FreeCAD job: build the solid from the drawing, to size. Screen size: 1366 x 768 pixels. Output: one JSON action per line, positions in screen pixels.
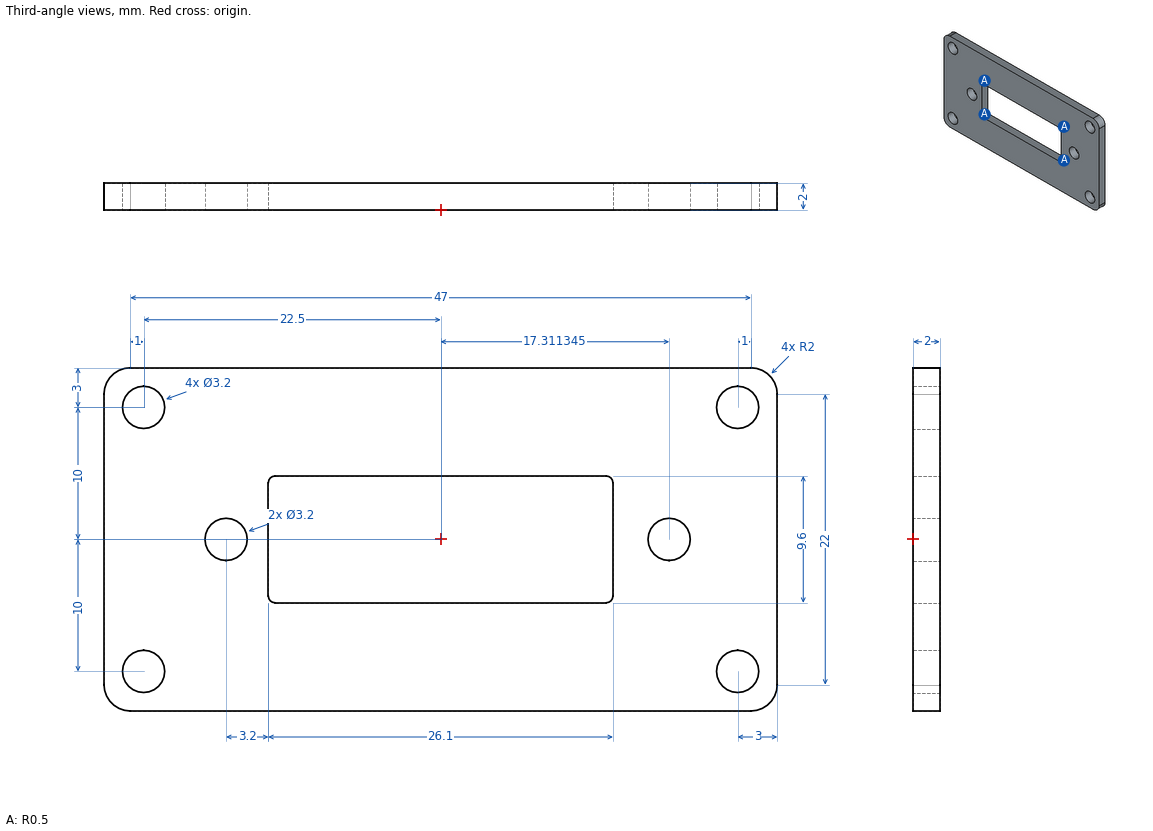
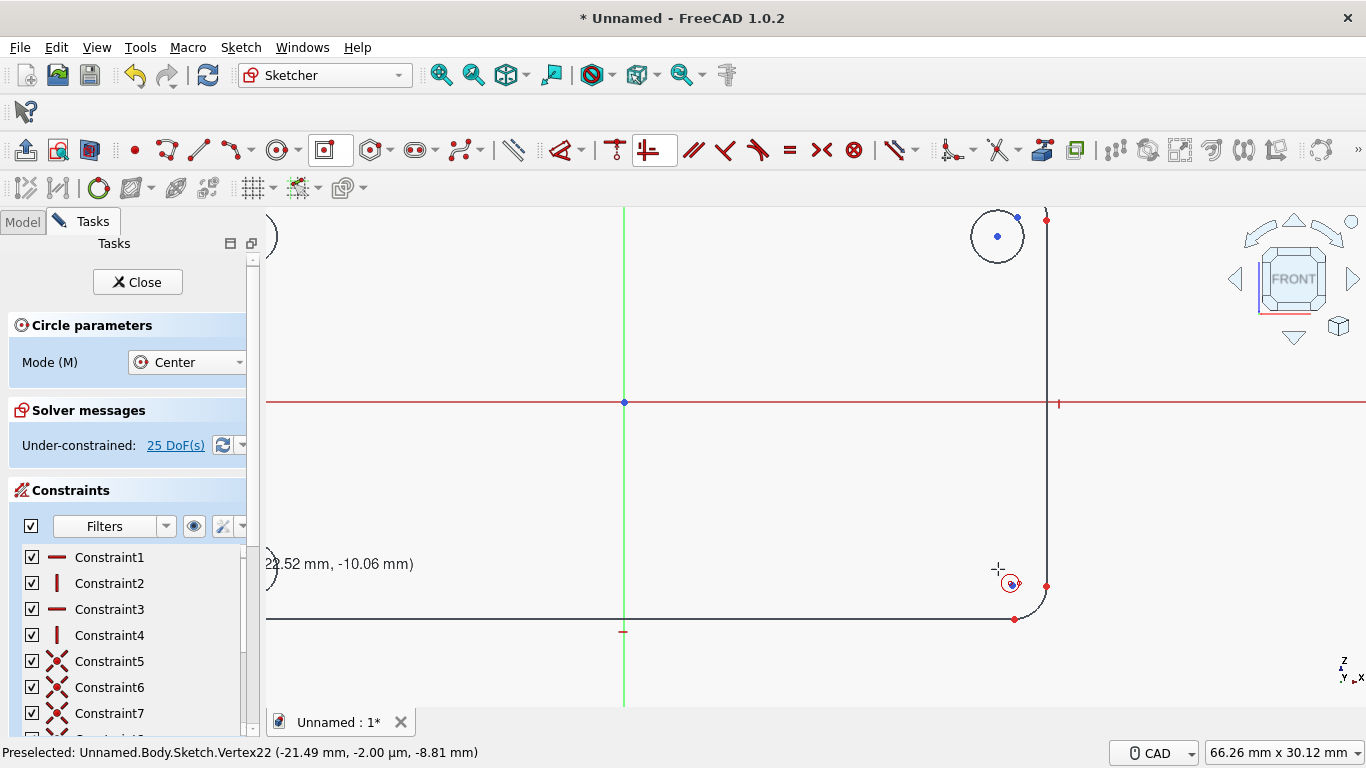
{"action": "left_click", "coordinate": [998, 568]}
{"action": "left_click", "coordinate": [1016, 549]}
{"action": "key", "text": "Escape"}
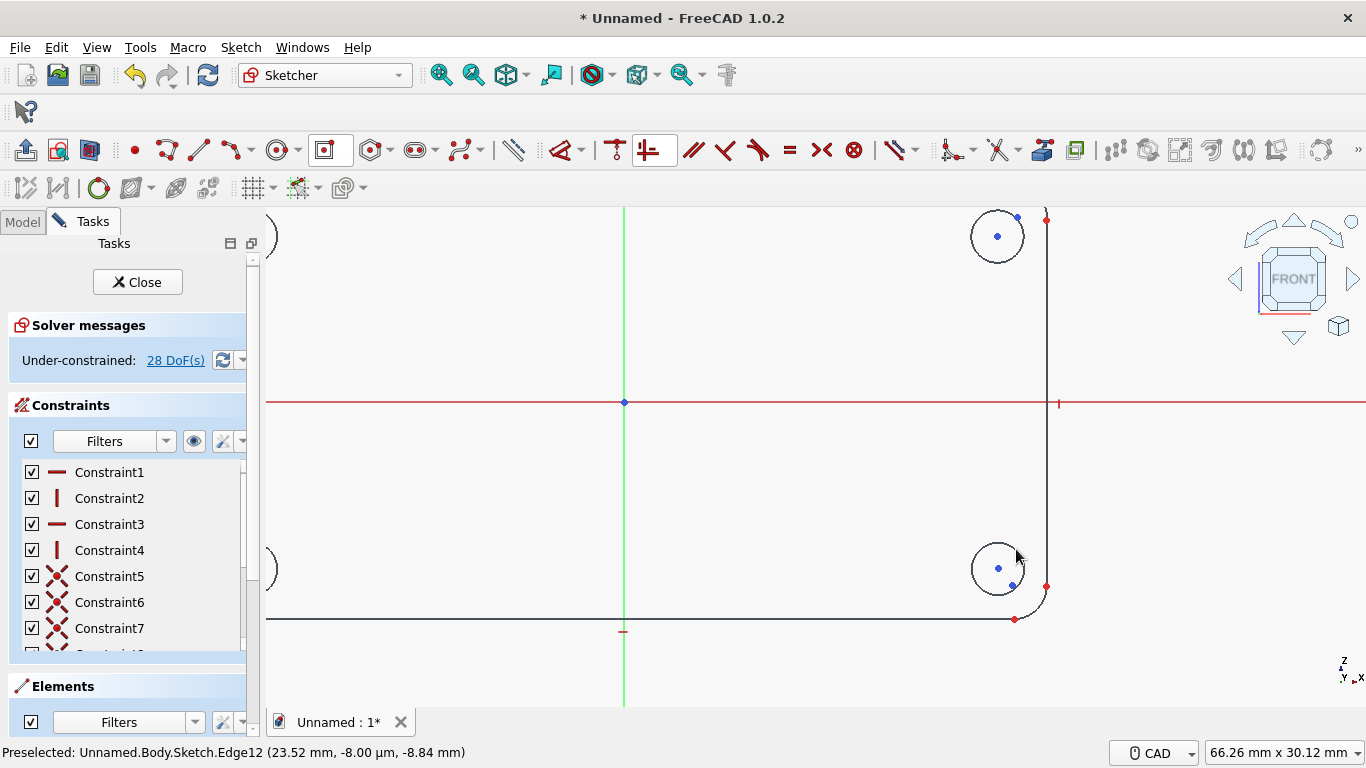
{"action": "scroll", "coordinate": [998, 569], "scroll_direction": "down", "scroll_amount": 2}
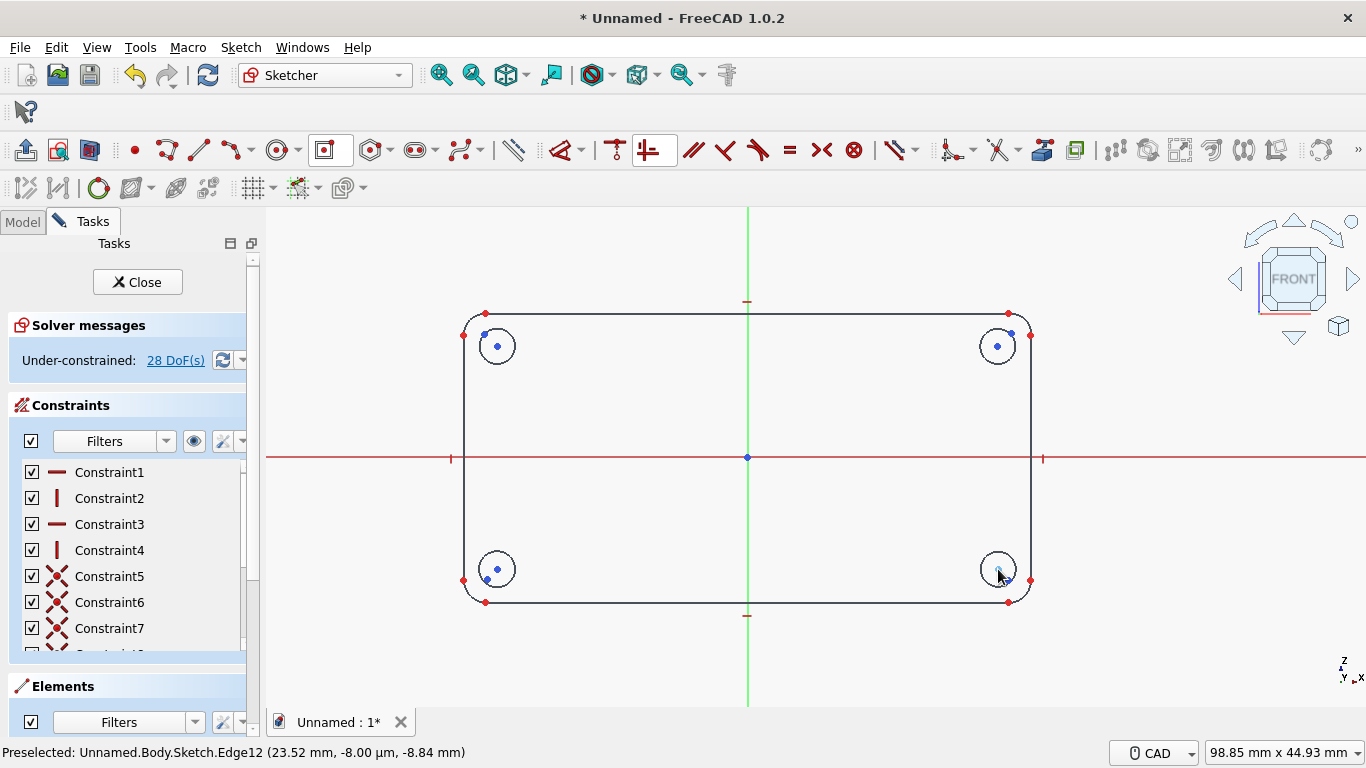
{"action": "left_click", "coordinate": [643, 314]}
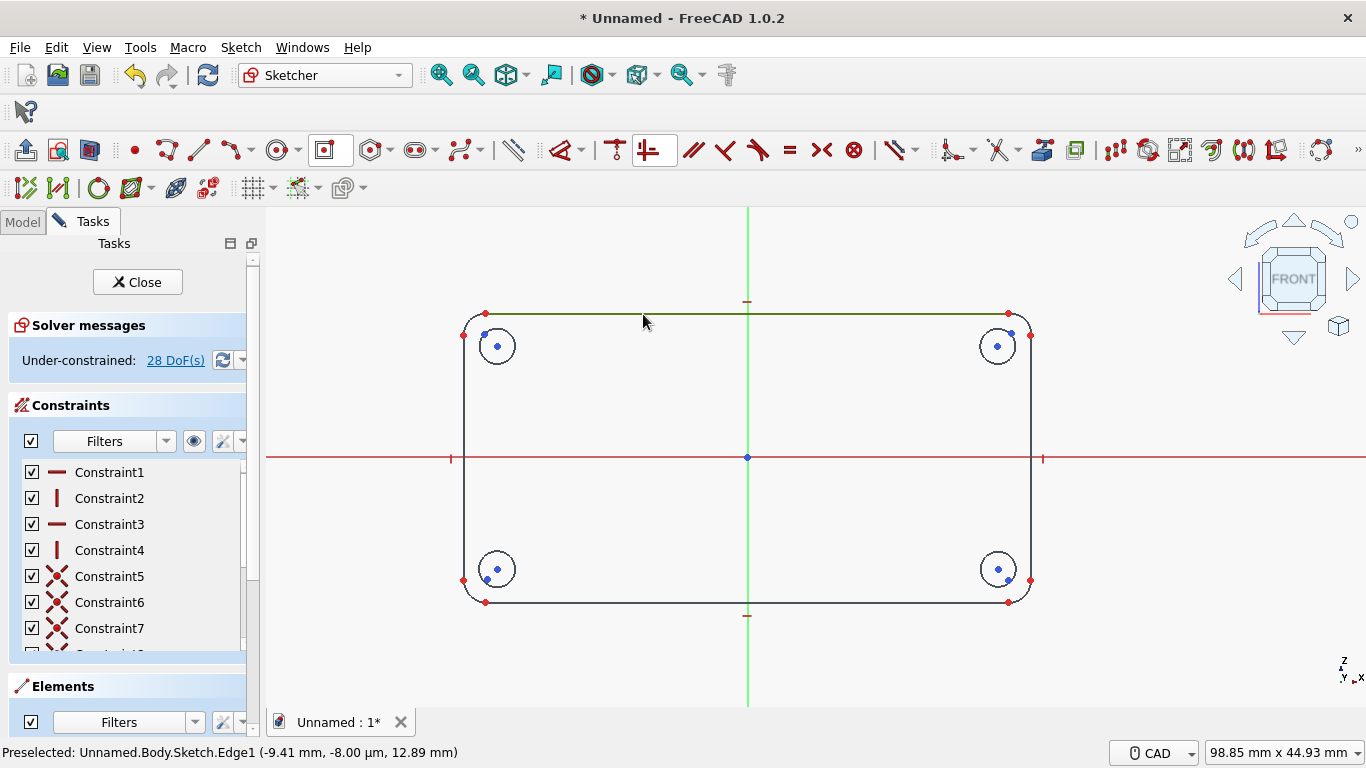
{"action": "scroll", "coordinate": [1029, 326], "scroll_direction": "up", "scroll_amount": 2}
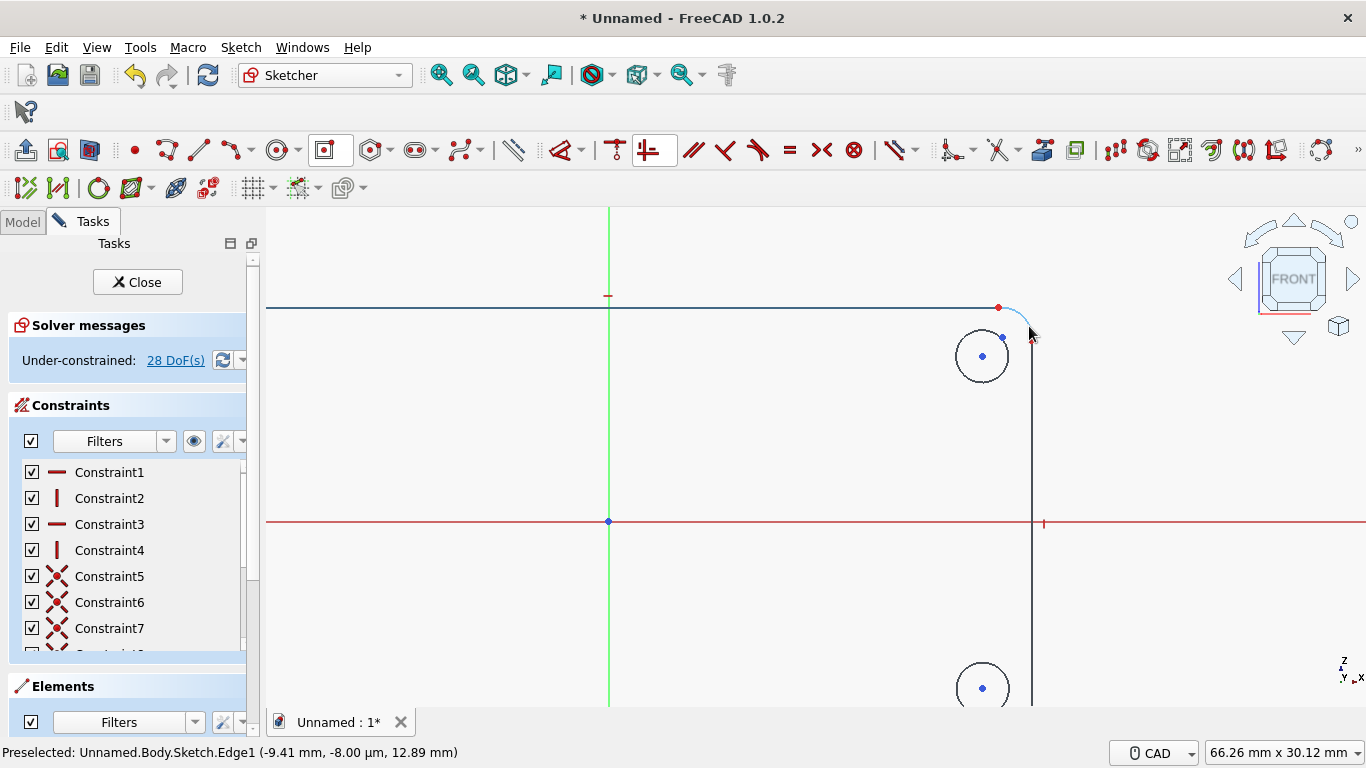
{"action": "left_click", "coordinate": [1029, 325]}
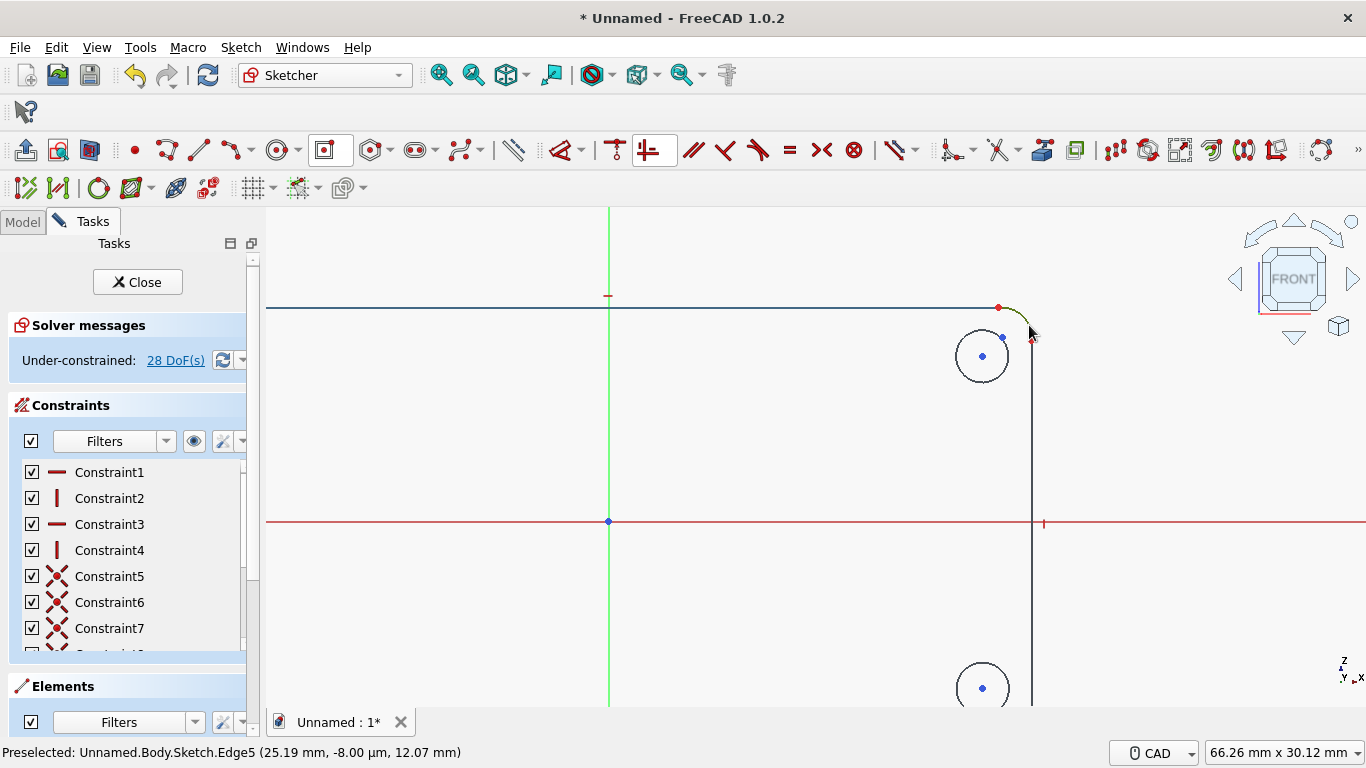
{"action": "left_click", "coordinate": [758, 150]}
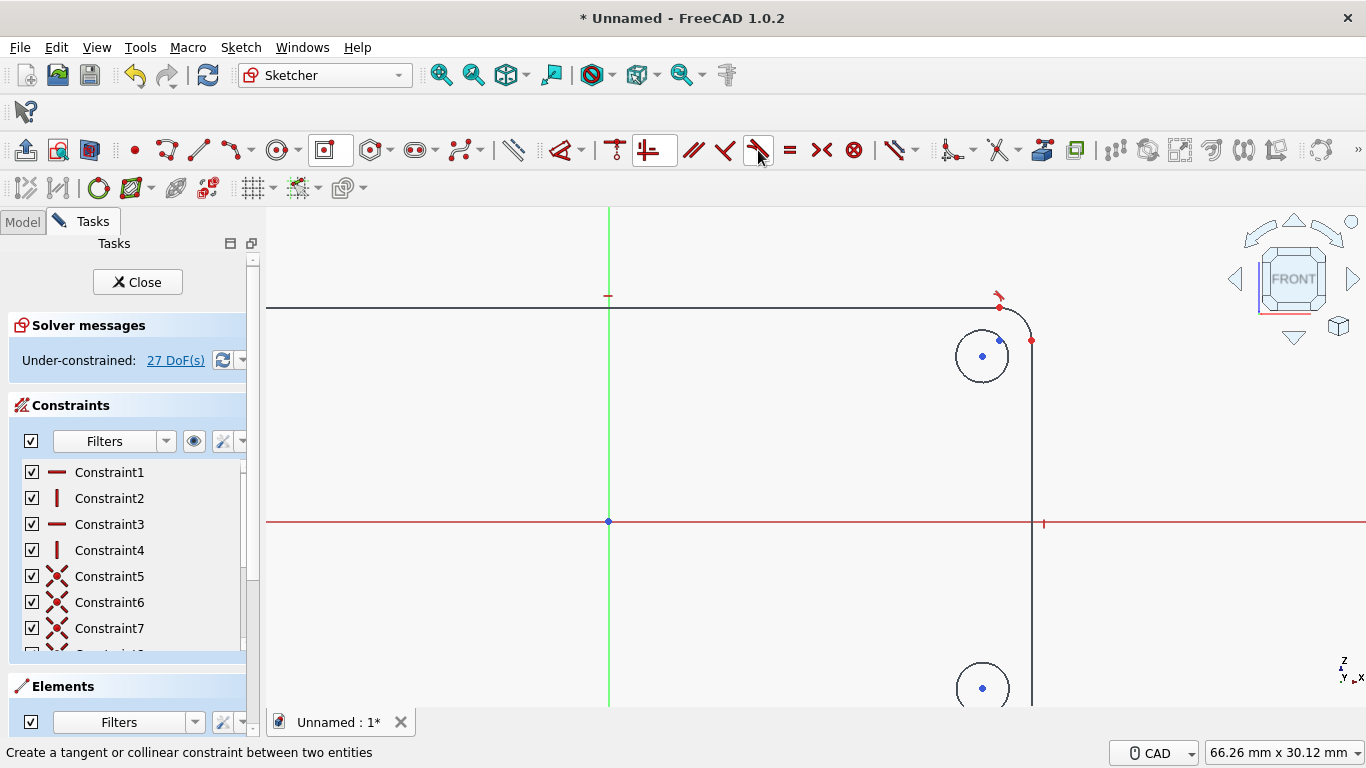
{"action": "left_click", "coordinate": [453, 308]}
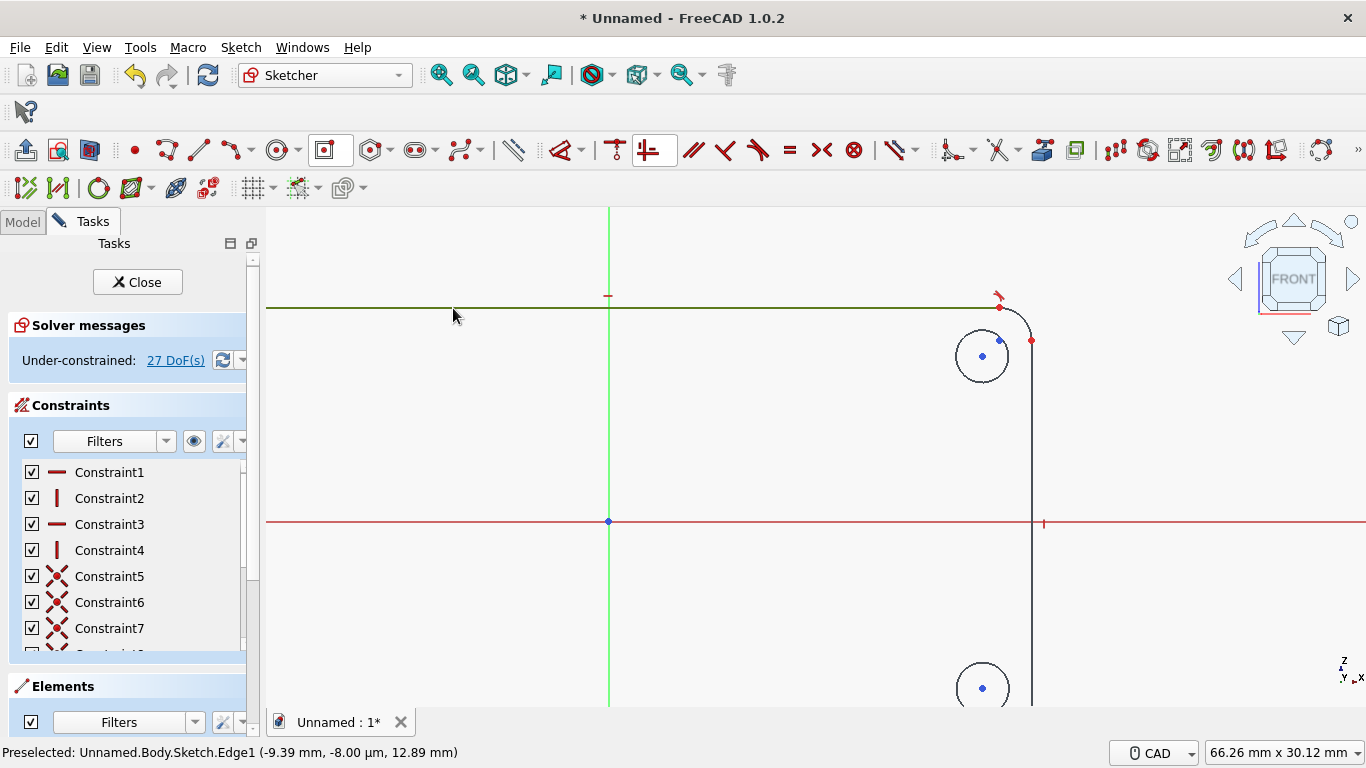
{"action": "scroll", "coordinate": [1029, 325], "scroll_direction": "down", "scroll_amount": 2}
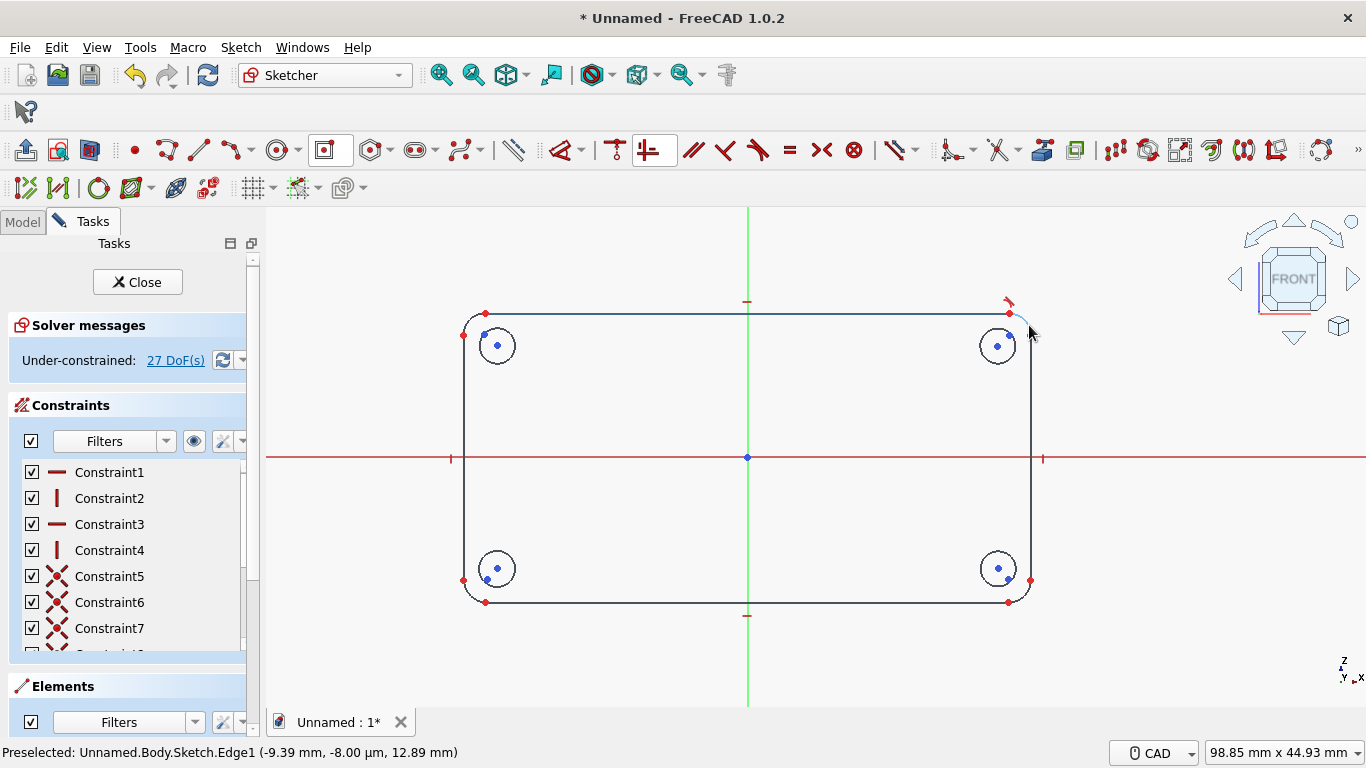
{"action": "scroll", "coordinate": [476, 316], "scroll_direction": "up", "scroll_amount": 2}